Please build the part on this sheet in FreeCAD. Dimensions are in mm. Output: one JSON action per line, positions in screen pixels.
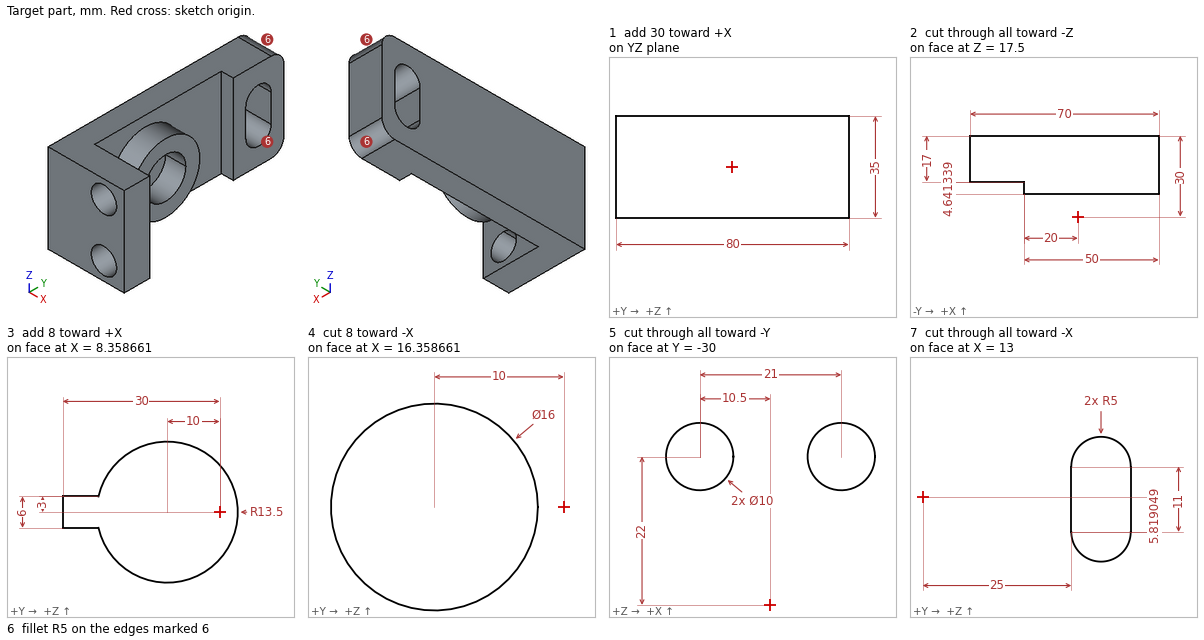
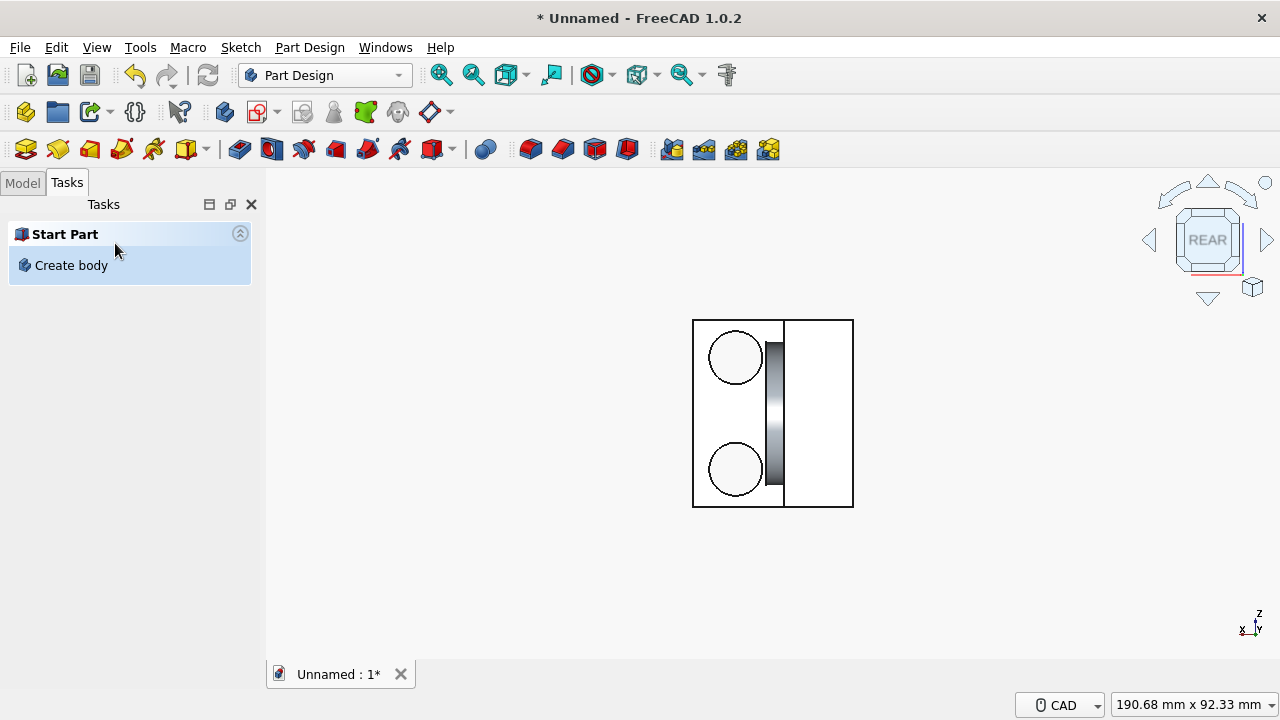
{"action": "key", "text": "v f"}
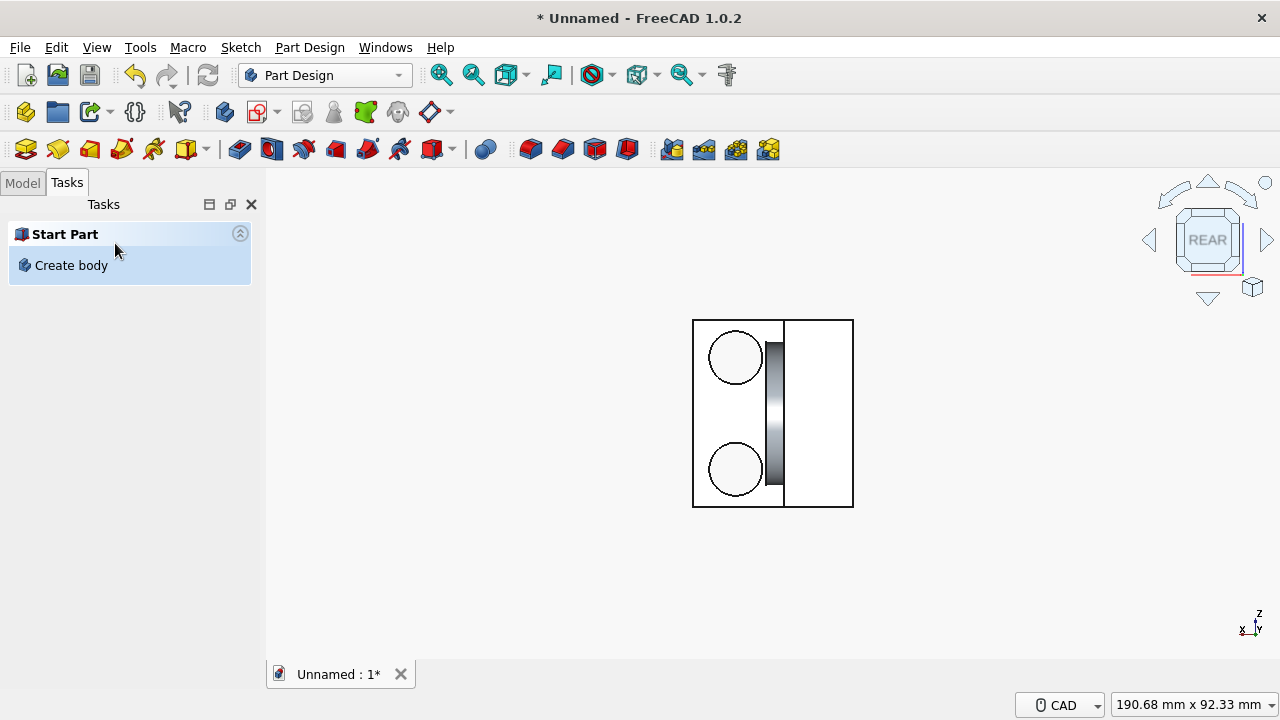
{"action": "left_click", "coordinate": [818, 319]}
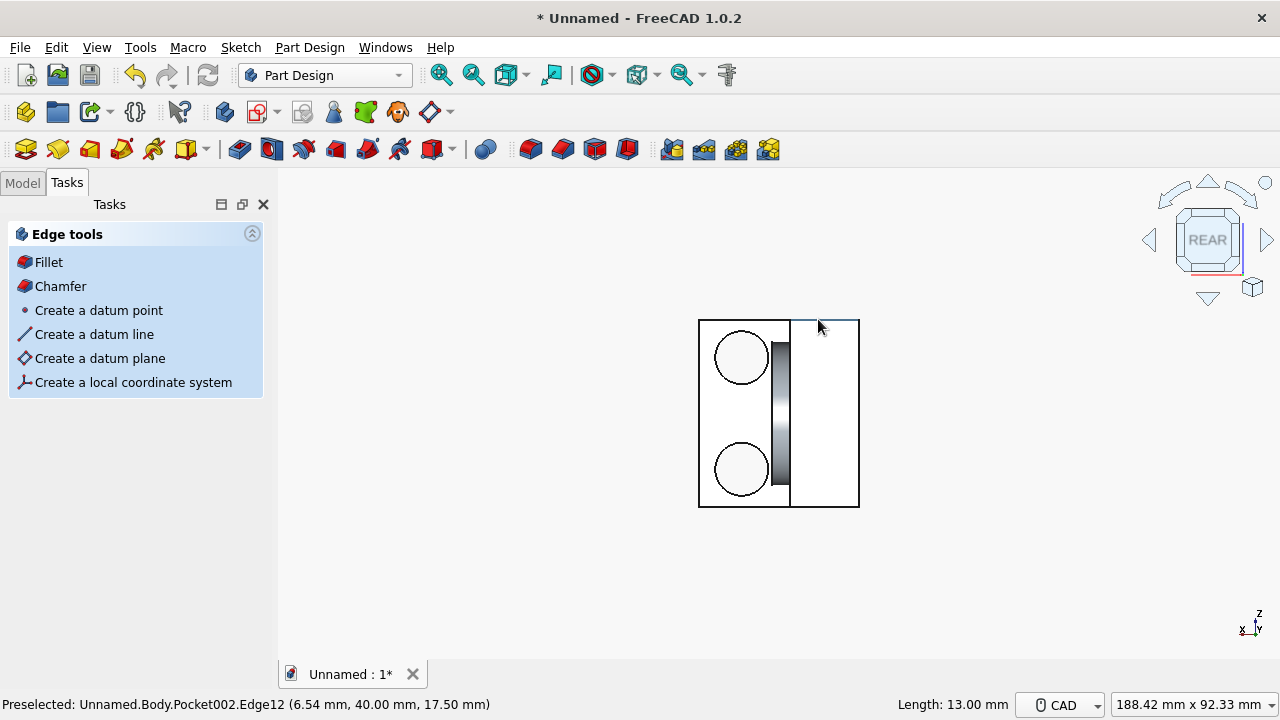
{"action": "left_click", "coordinate": [824, 506], "text": "ctrl"}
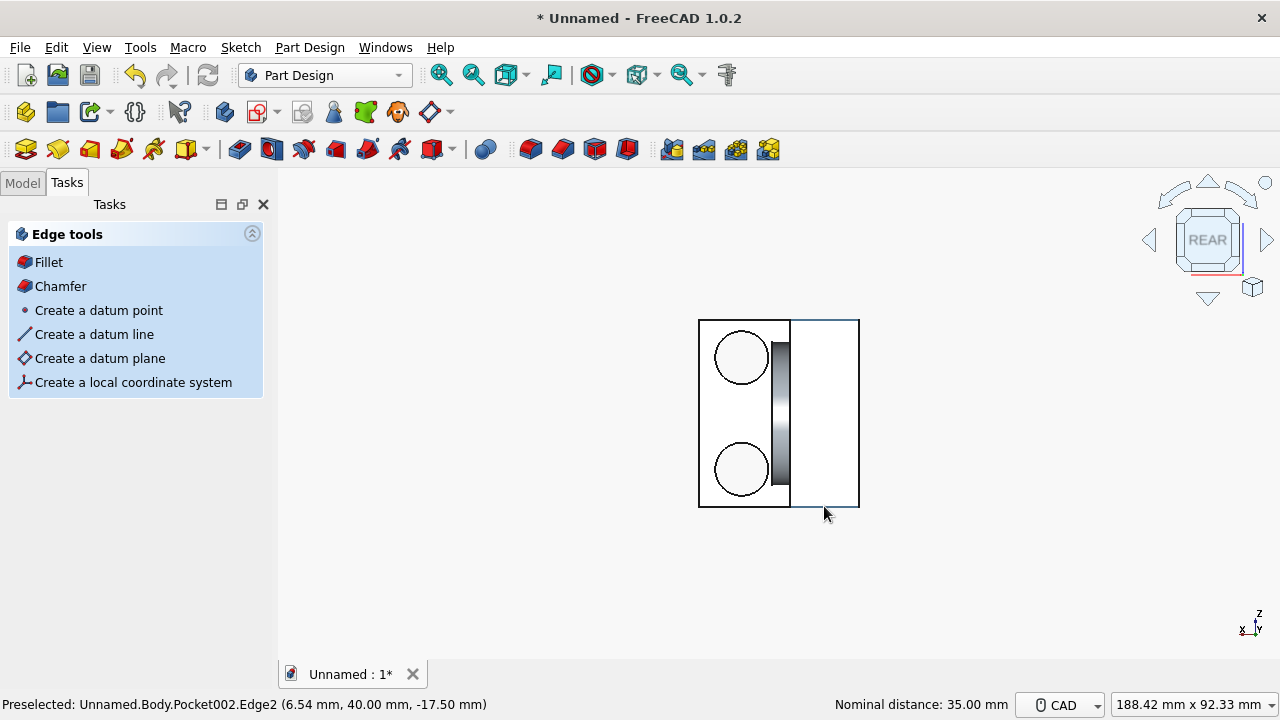
{"action": "left_click", "coordinate": [532, 150]}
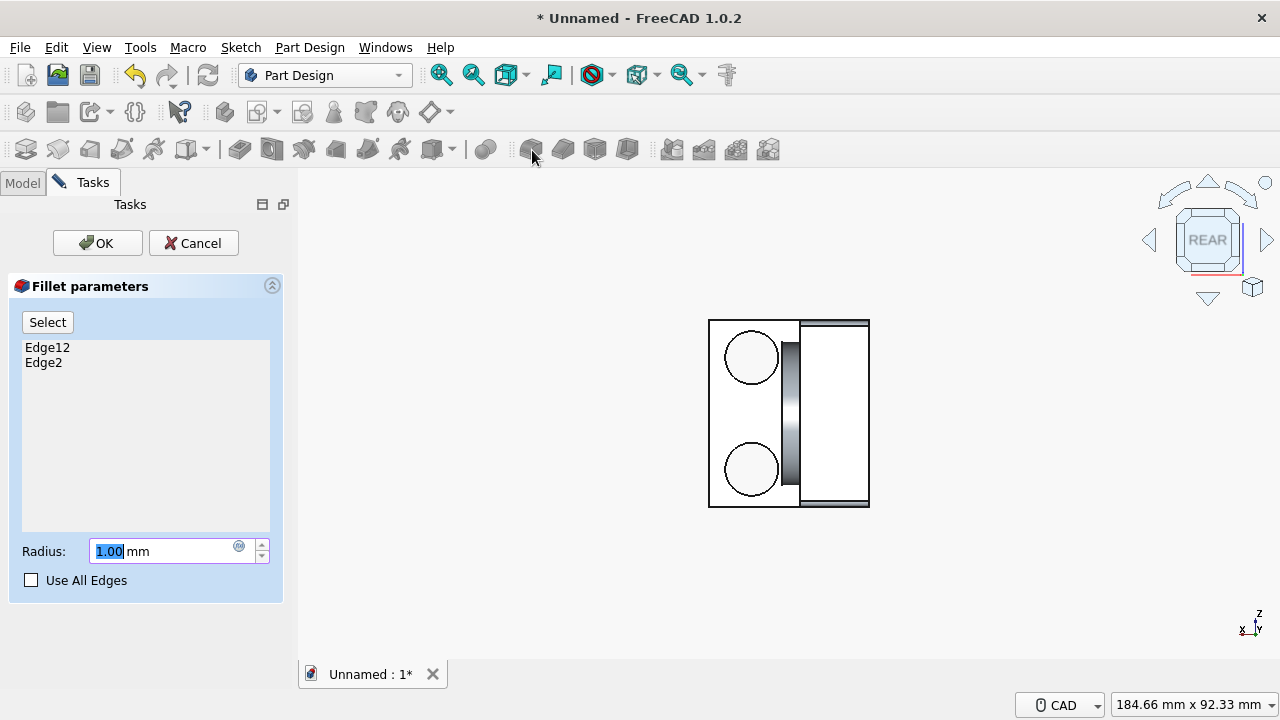
{"action": "type", "text": "5"}
{"action": "key", "text": "Tab"}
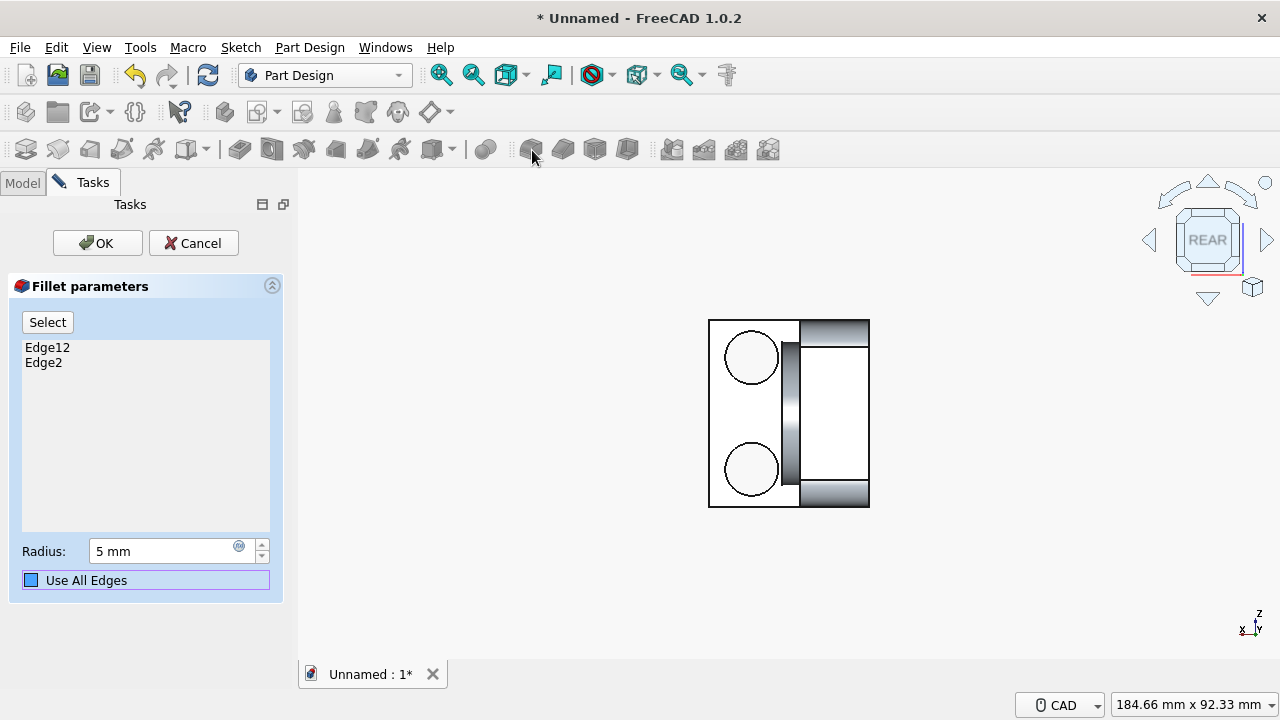
{"action": "left_click", "coordinate": [98, 243]}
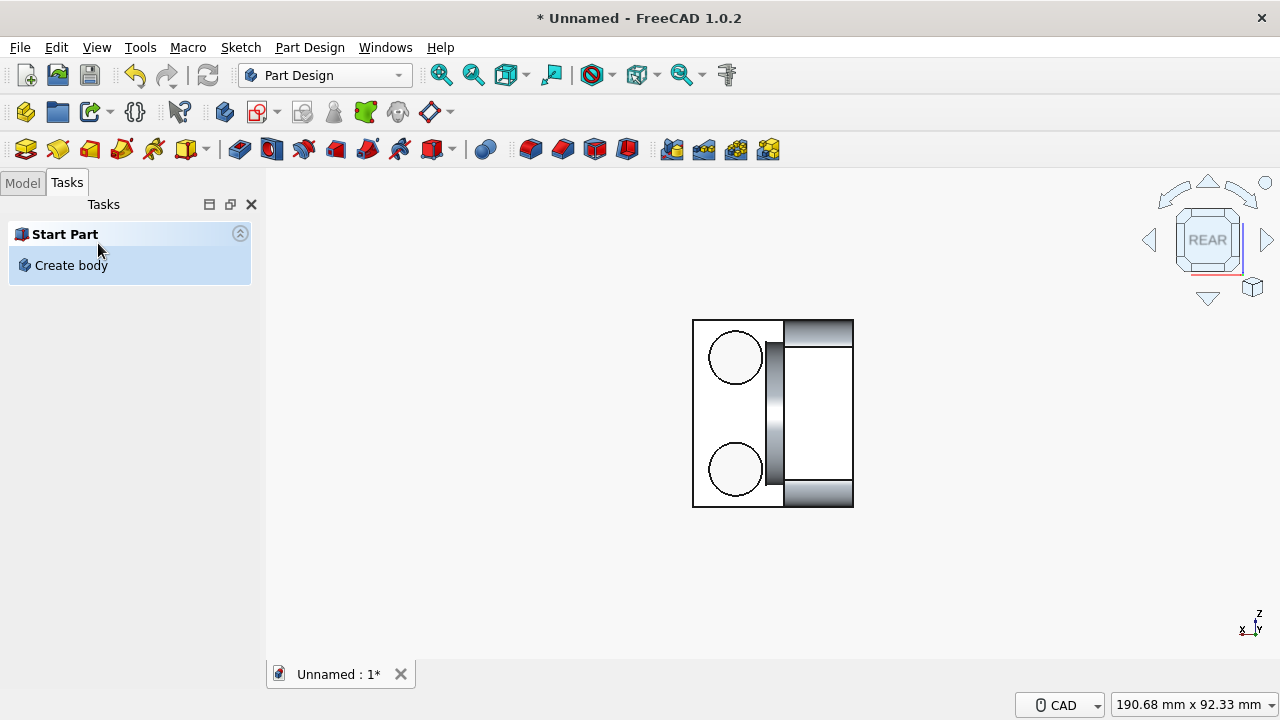
{"action": "left_click", "coordinate": [442, 76]}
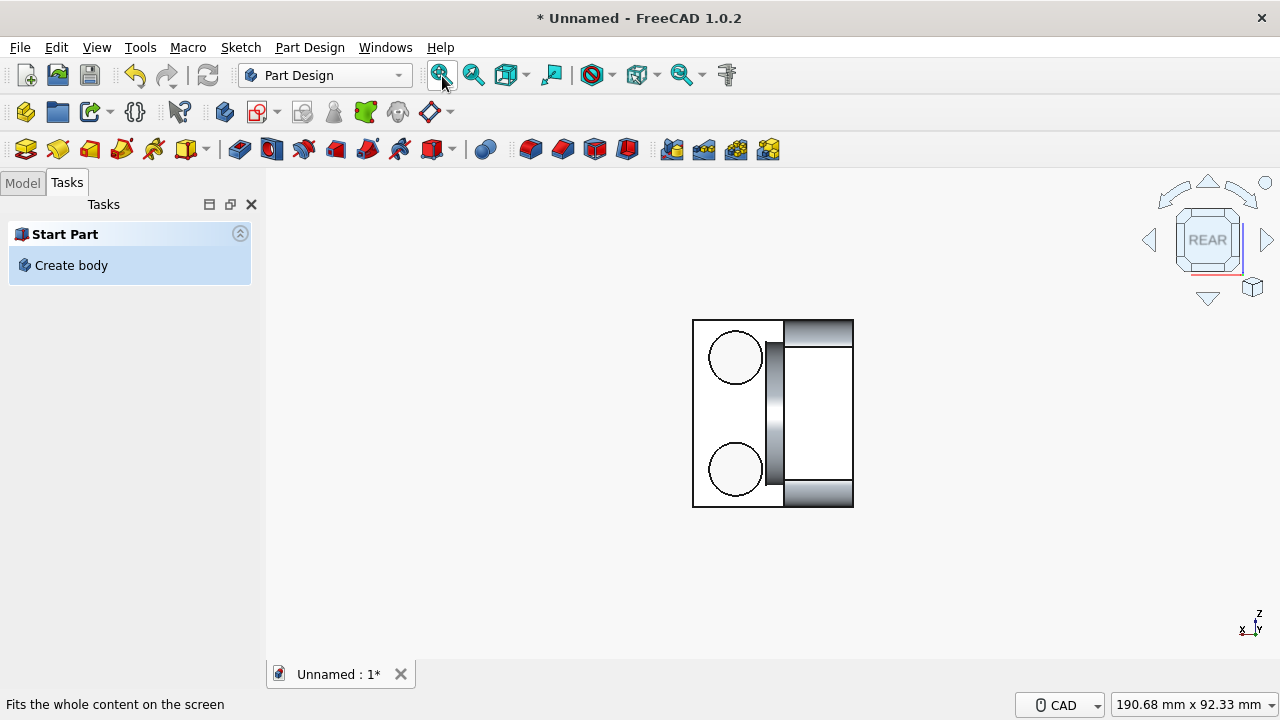
{"action": "key", "text": "0"}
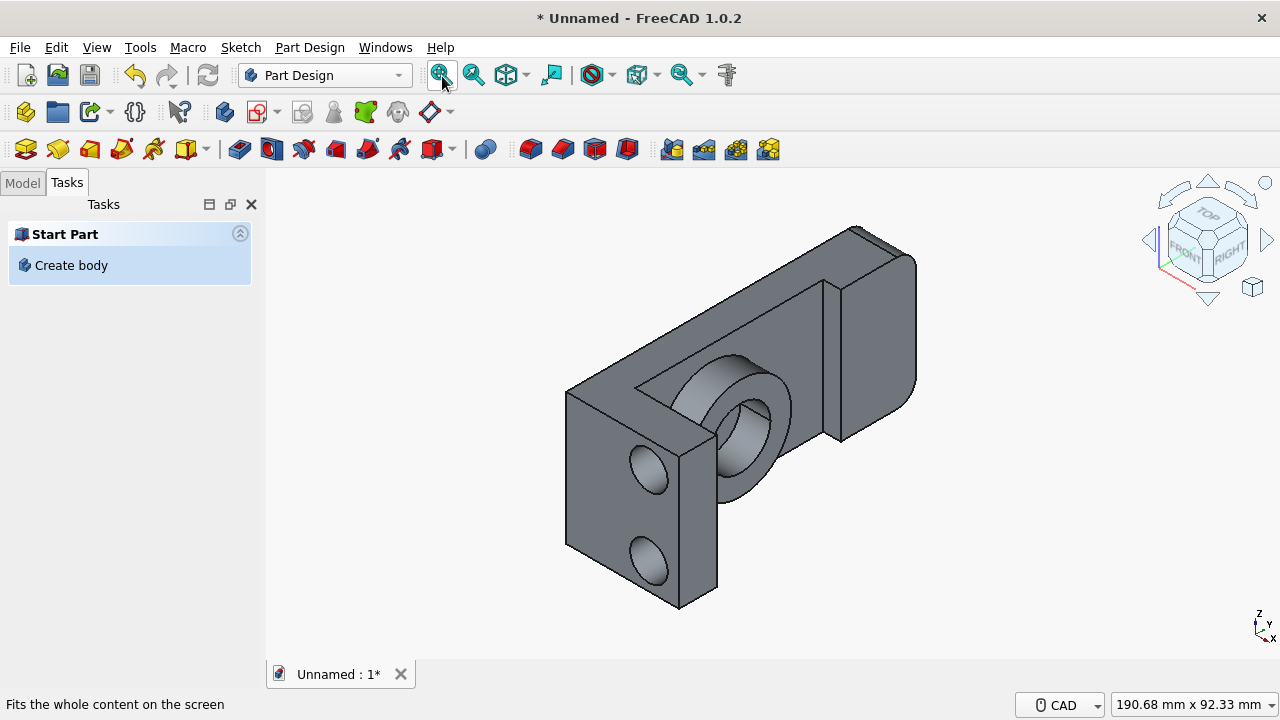
{"action": "left_click", "coordinate": [878, 365]}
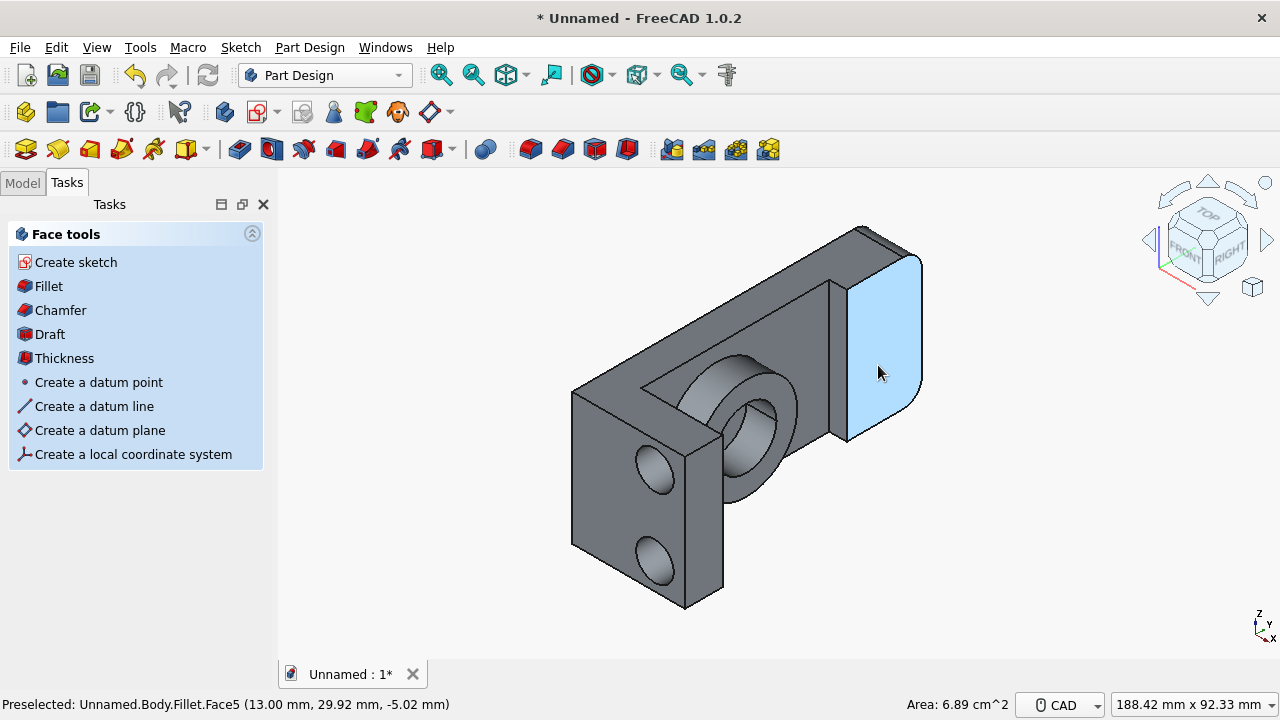
{"action": "left_click", "coordinate": [258, 112]}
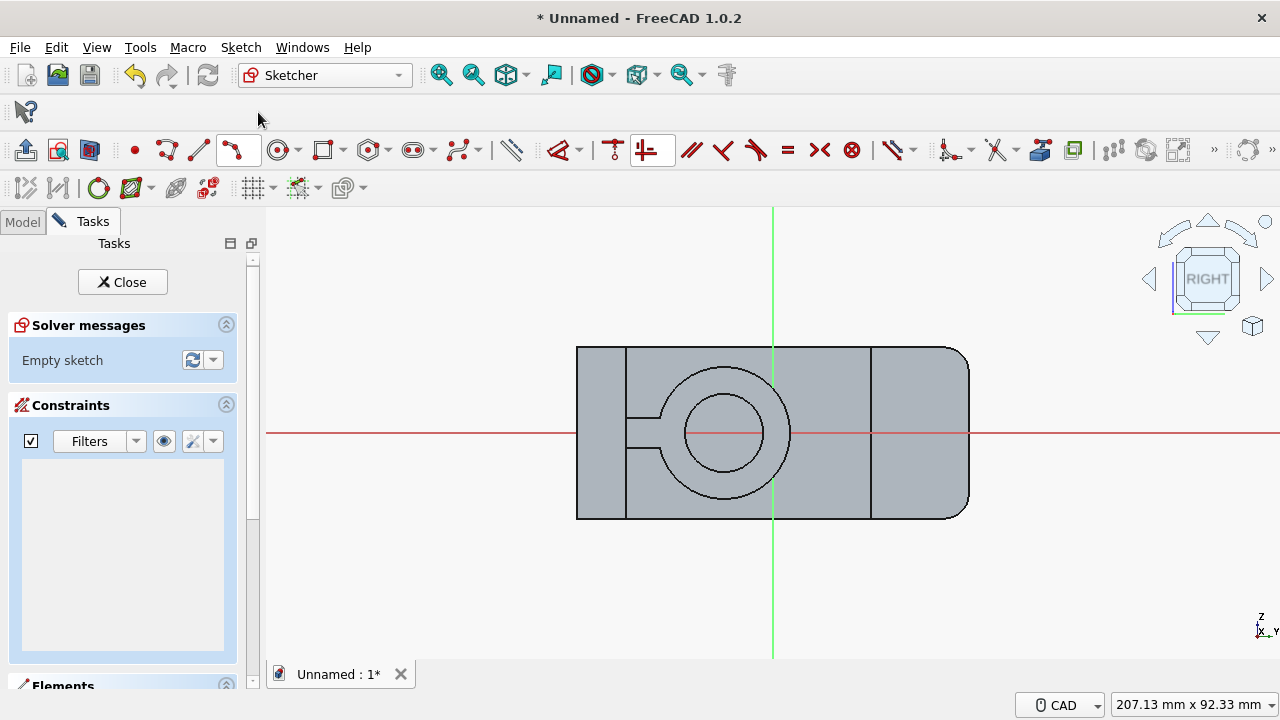
{"action": "scroll", "coordinate": [948, 435], "scroll_direction": "up", "scroll_amount": 5}